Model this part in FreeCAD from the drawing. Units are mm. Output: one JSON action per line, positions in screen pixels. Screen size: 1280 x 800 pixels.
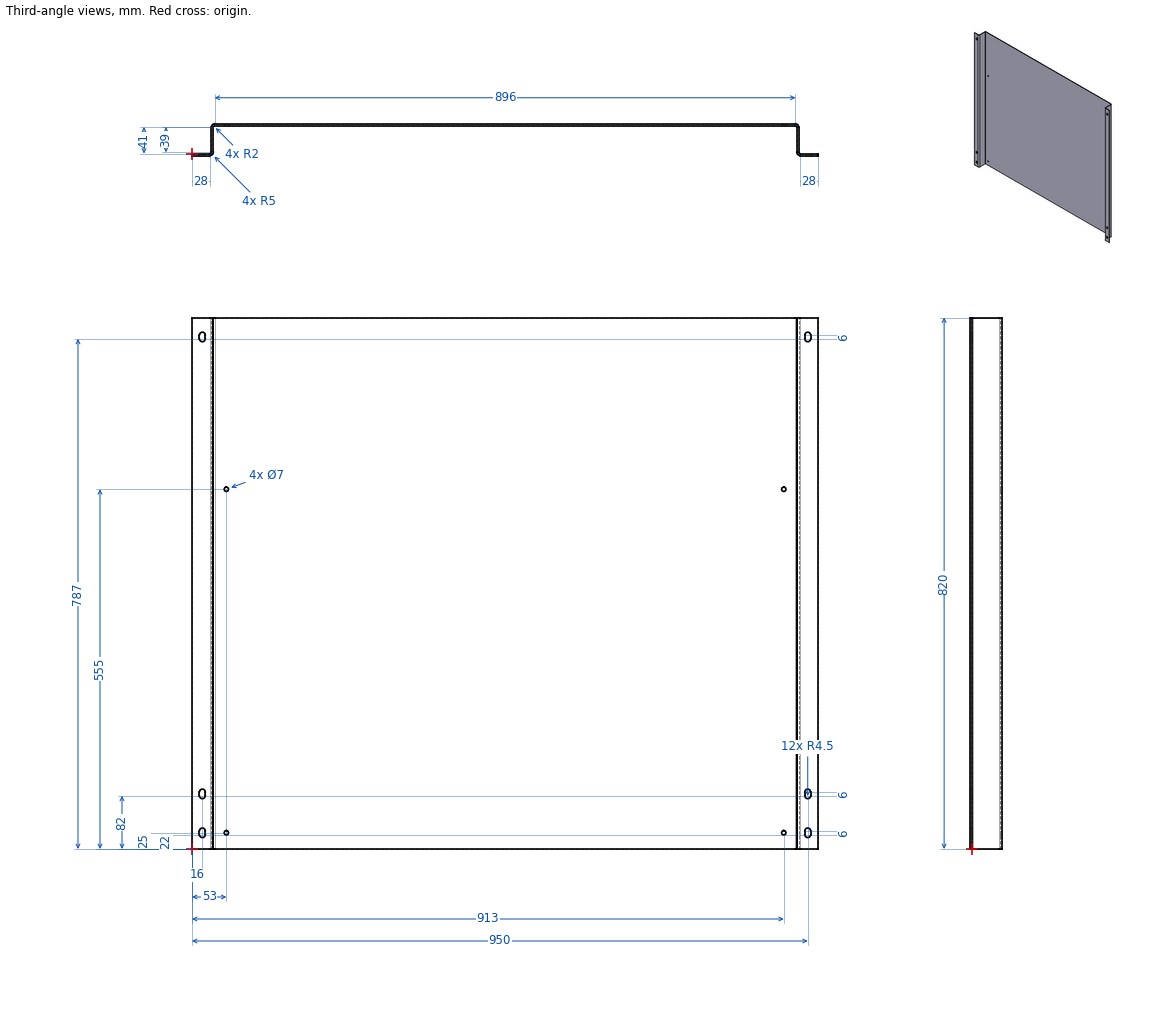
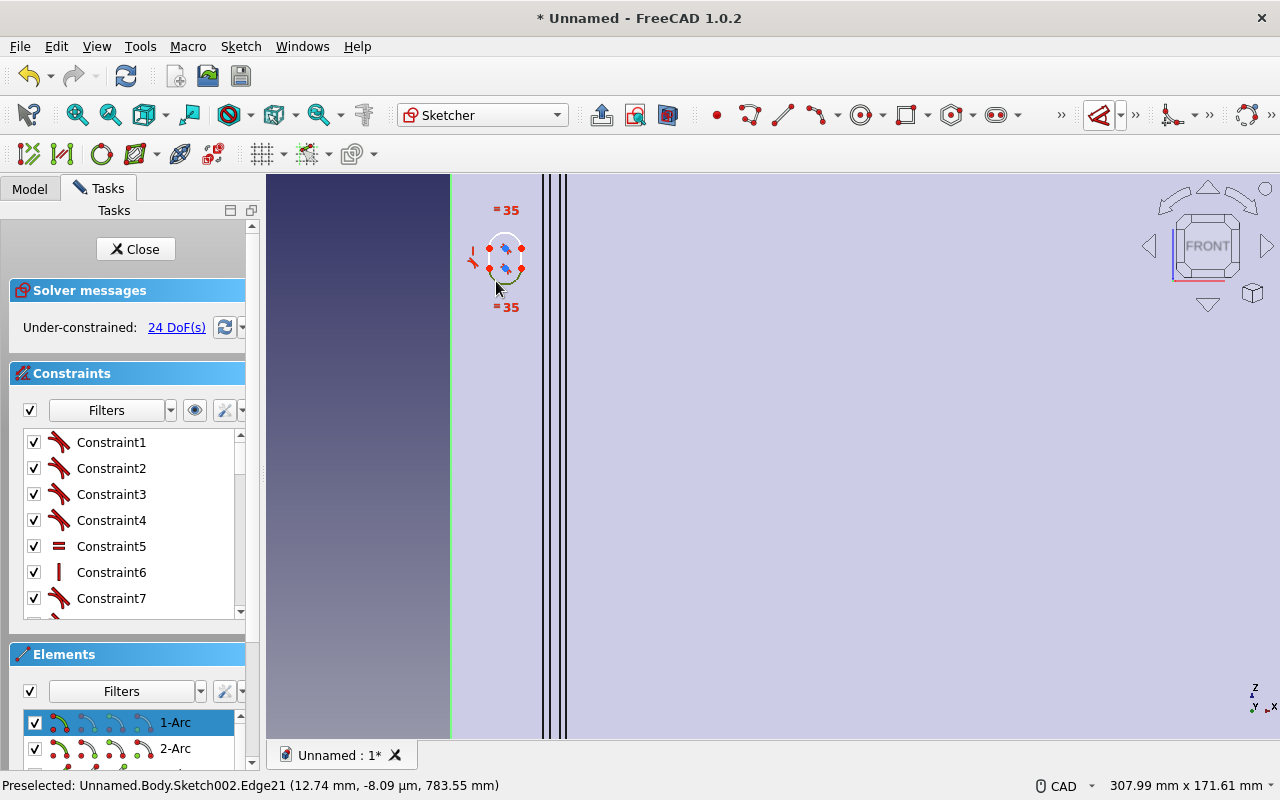
{"action": "key", "text": "e"}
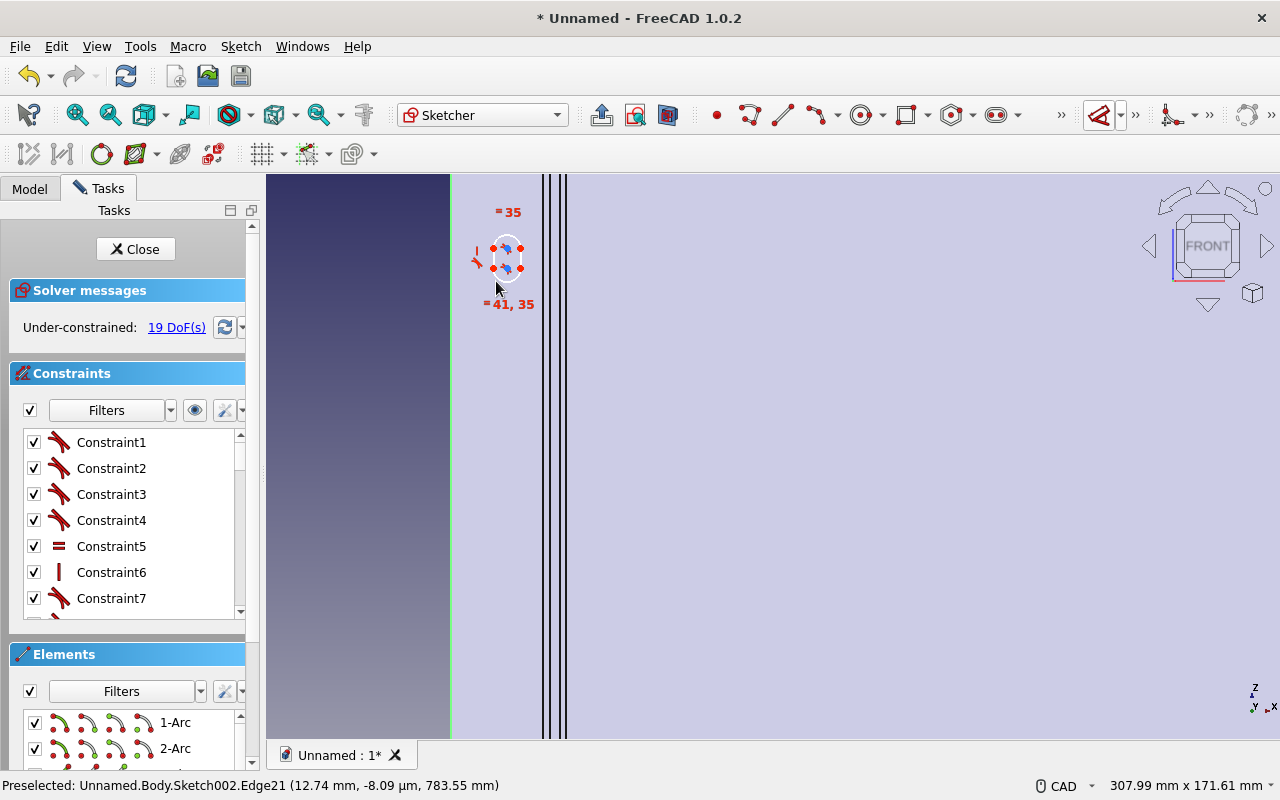
{"action": "key", "text": "d"}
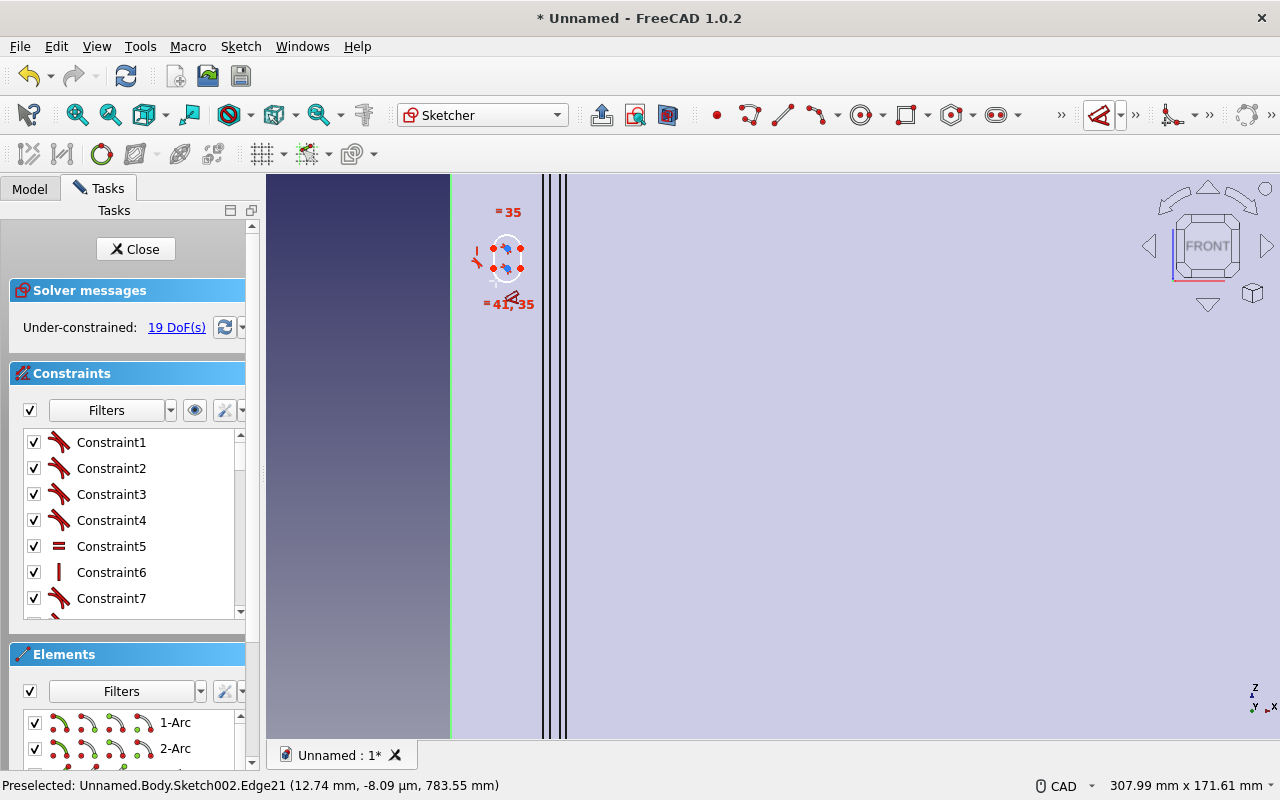
{"action": "scroll", "coordinate": [498, 286], "scroll_direction": "down", "scroll_amount": 10}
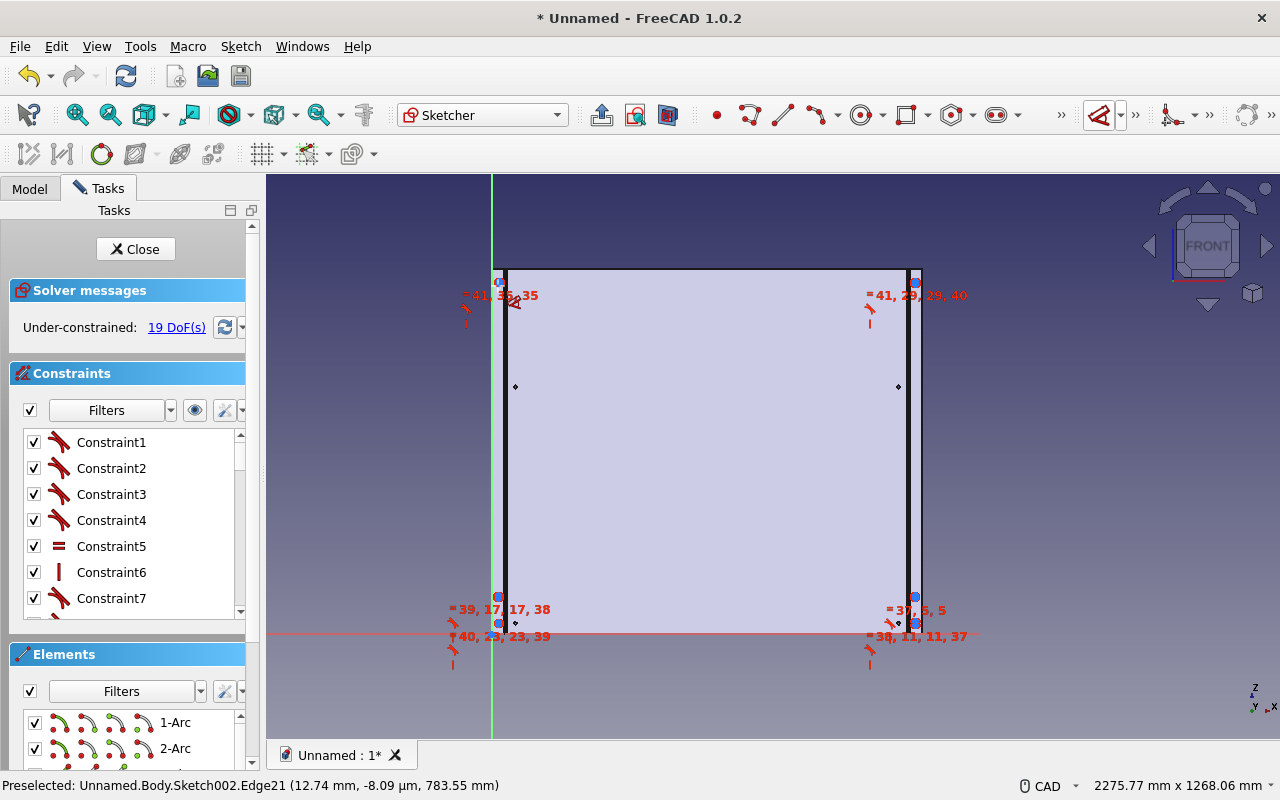
{"action": "scroll", "coordinate": [914, 600], "scroll_direction": "up", "scroll_amount": 15}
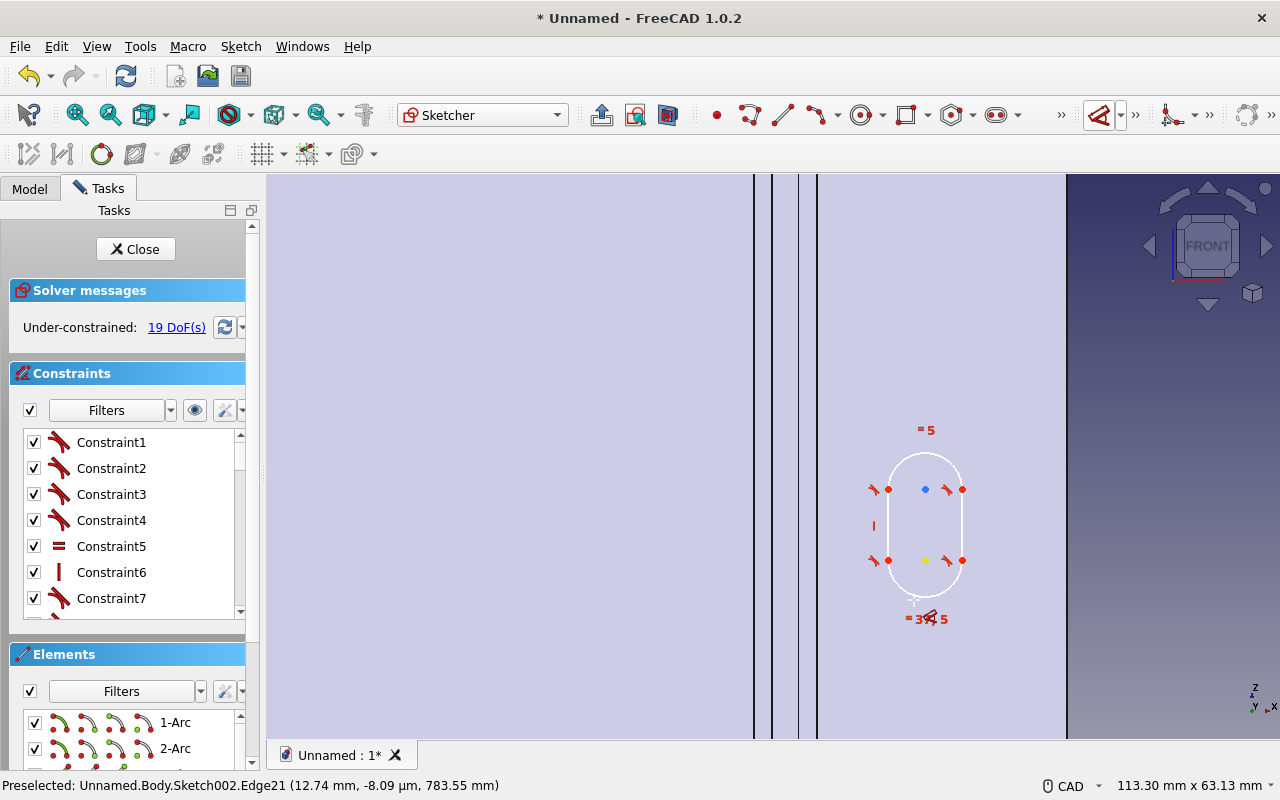
{"action": "left_click", "coordinate": [903, 590]}
{"action": "left_click", "coordinate": [884, 616]}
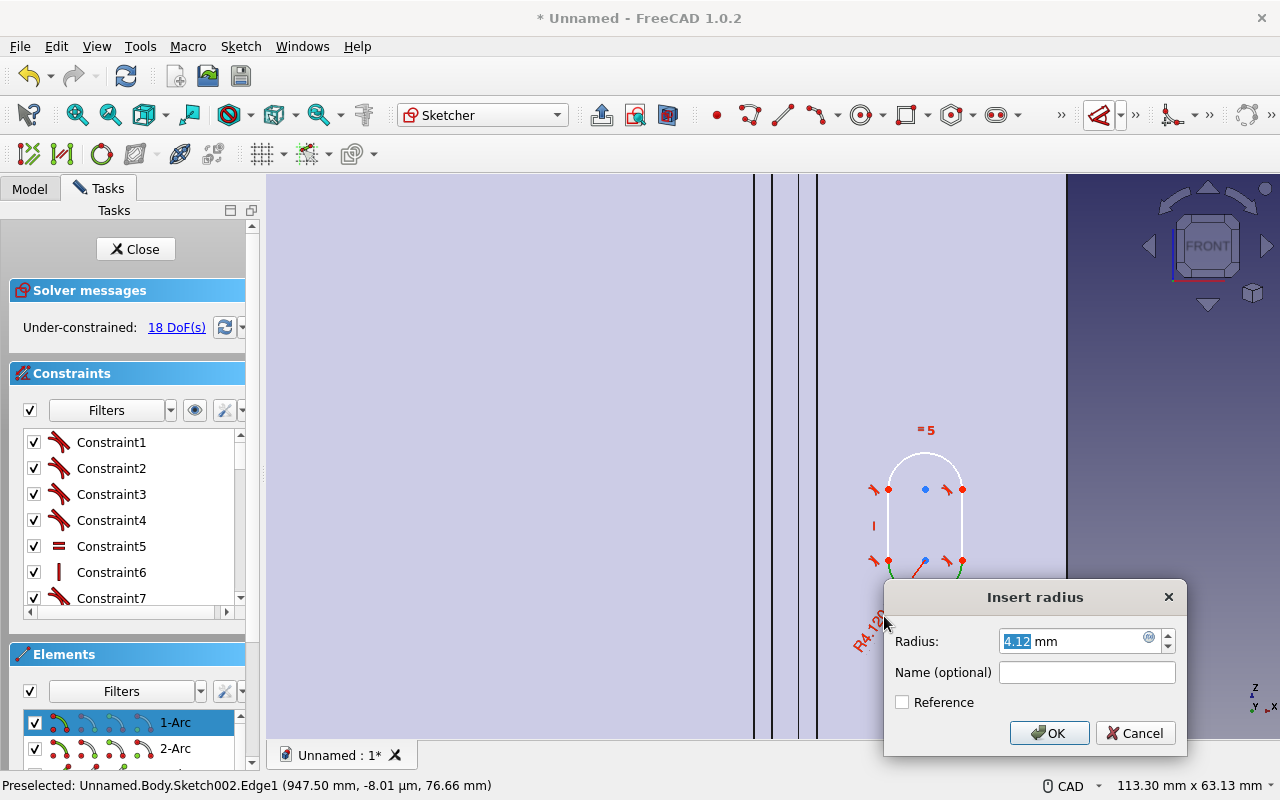
{"action": "type", "text": "4.5"}
{"action": "key", "text": "Return"}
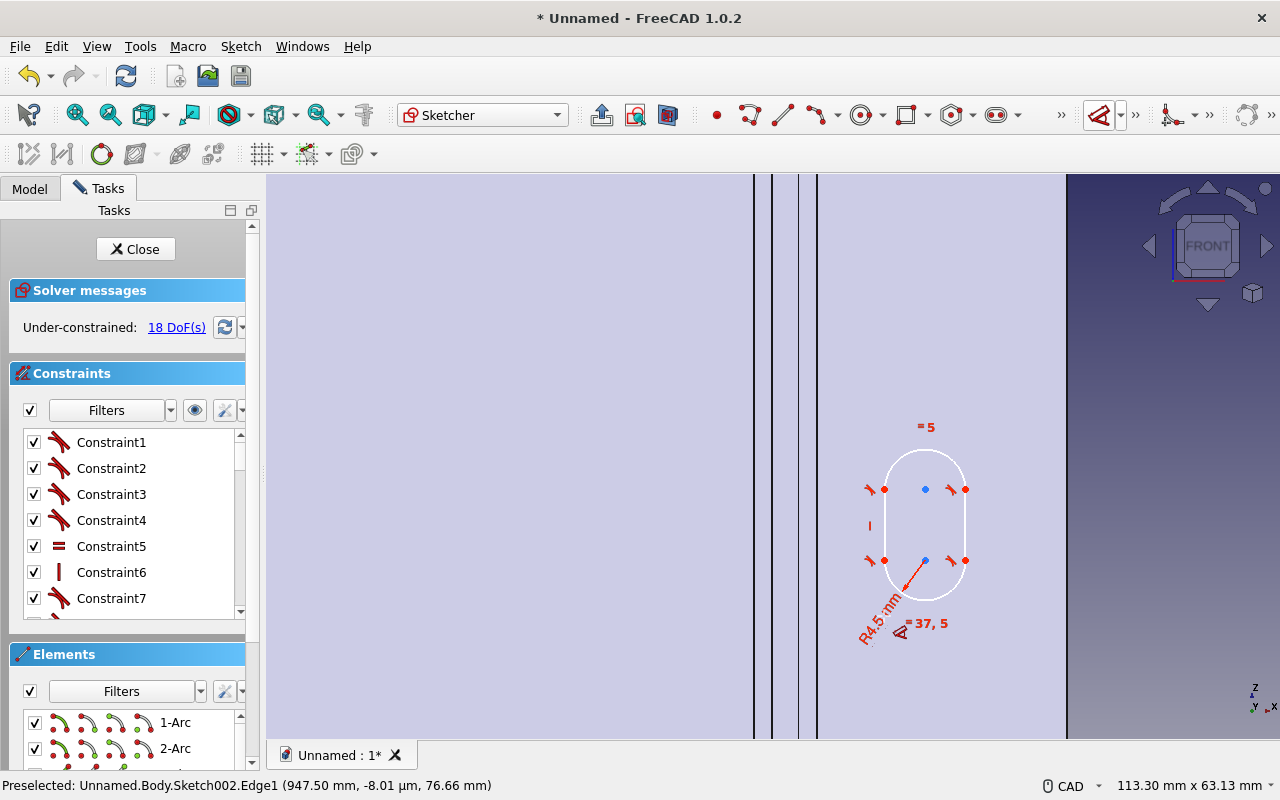
{"action": "left_click", "coordinate": [885, 539]}
{"action": "left_click", "coordinate": [919, 525]}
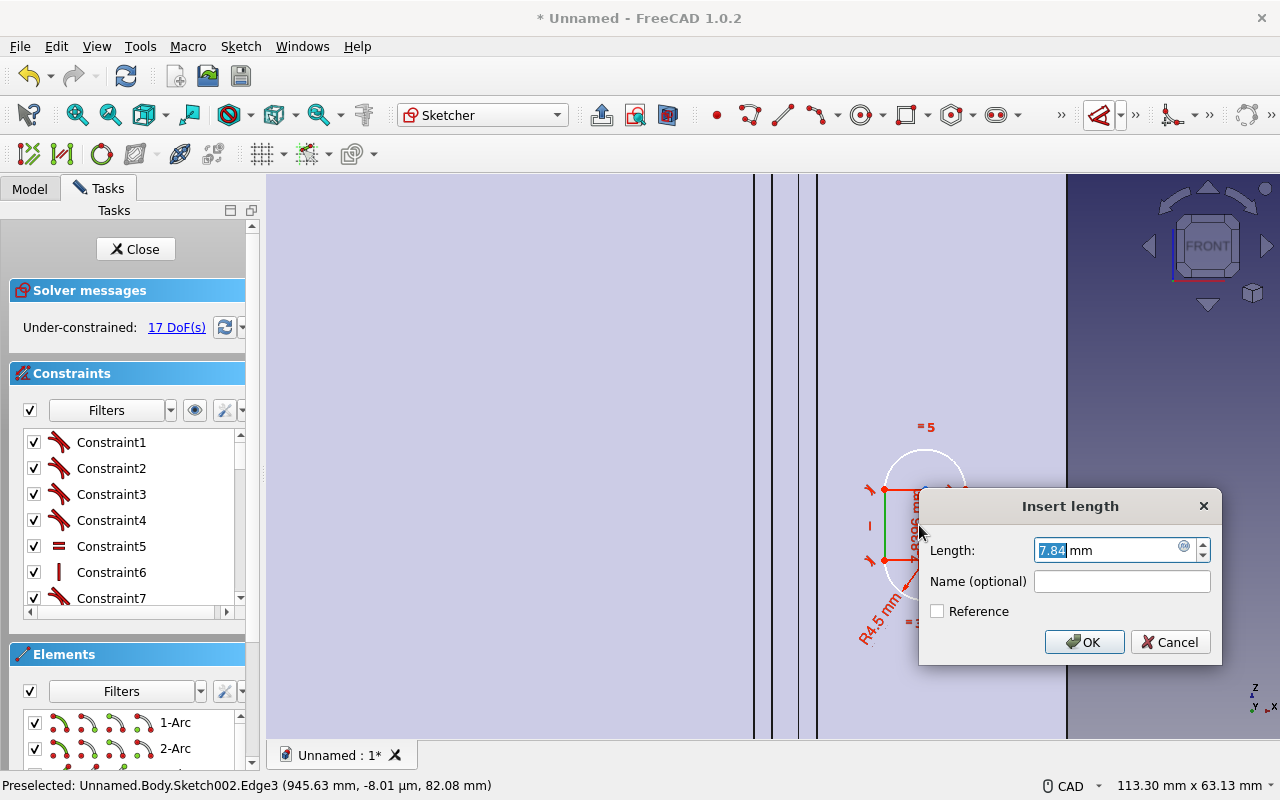
{"action": "type", "text": "6"}
{"action": "key", "text": "Return"}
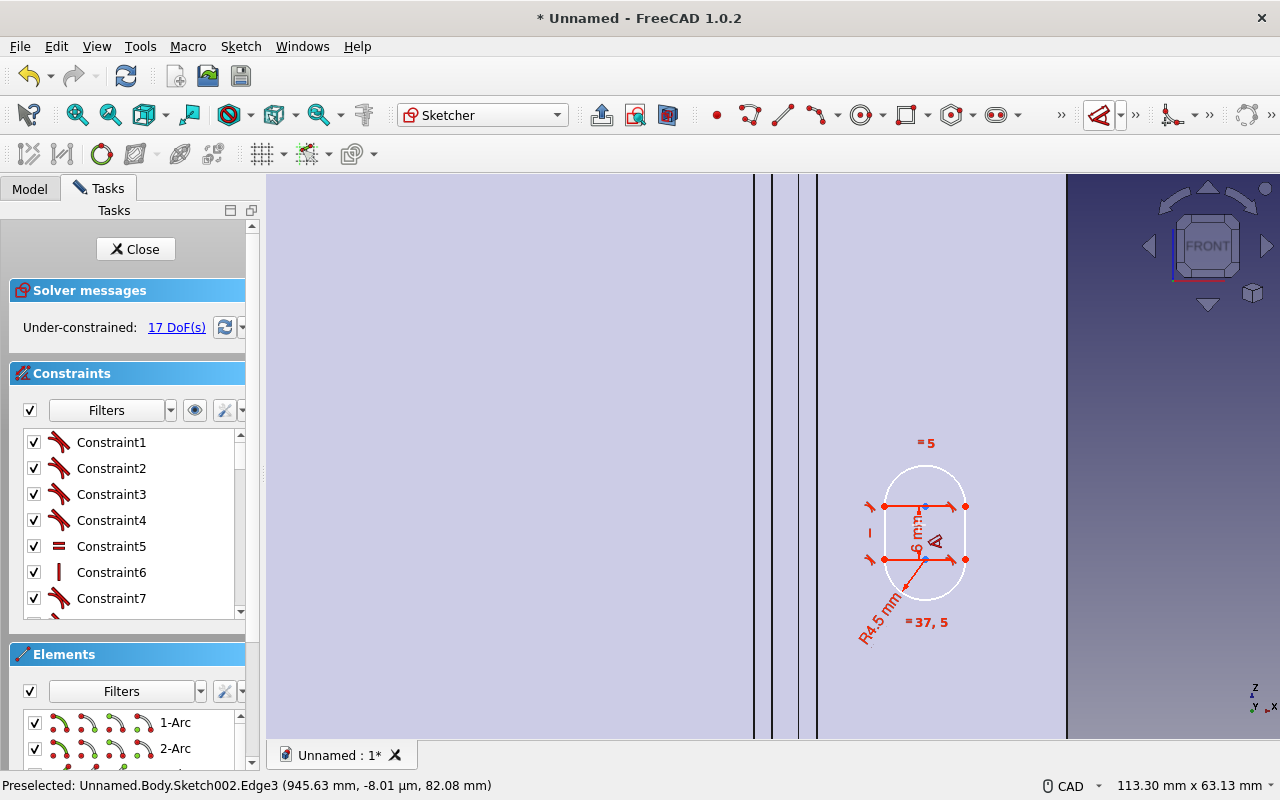
{"action": "scroll", "coordinate": [915, 601], "scroll_direction": "down", "scroll_amount": 15}